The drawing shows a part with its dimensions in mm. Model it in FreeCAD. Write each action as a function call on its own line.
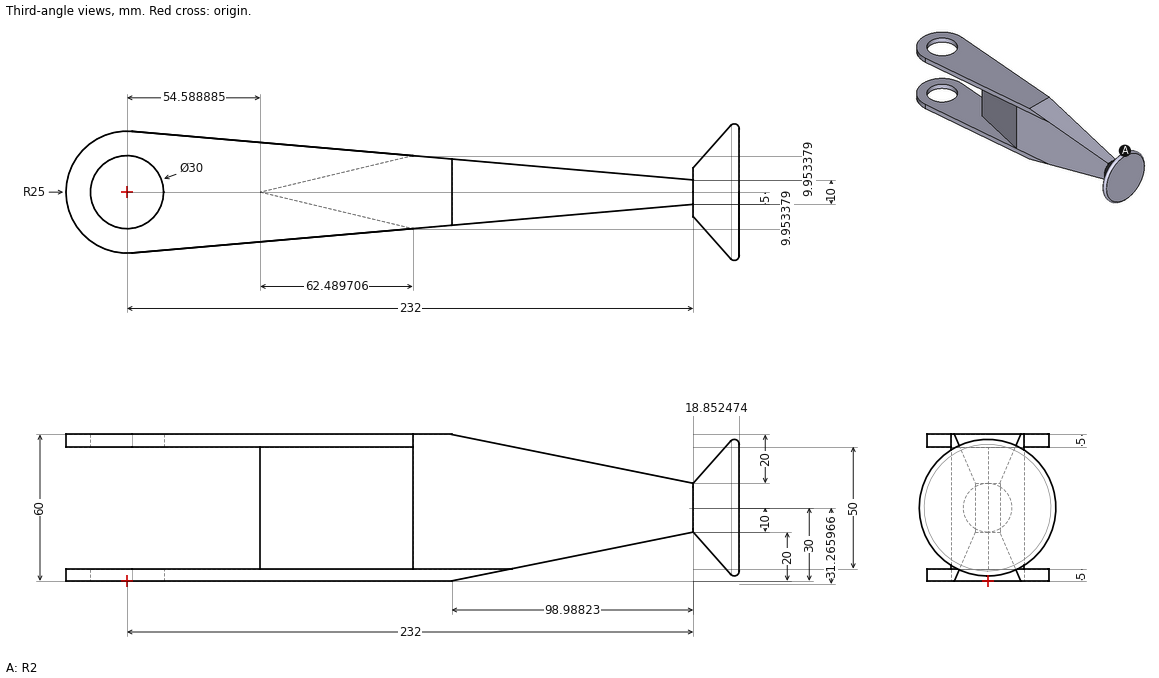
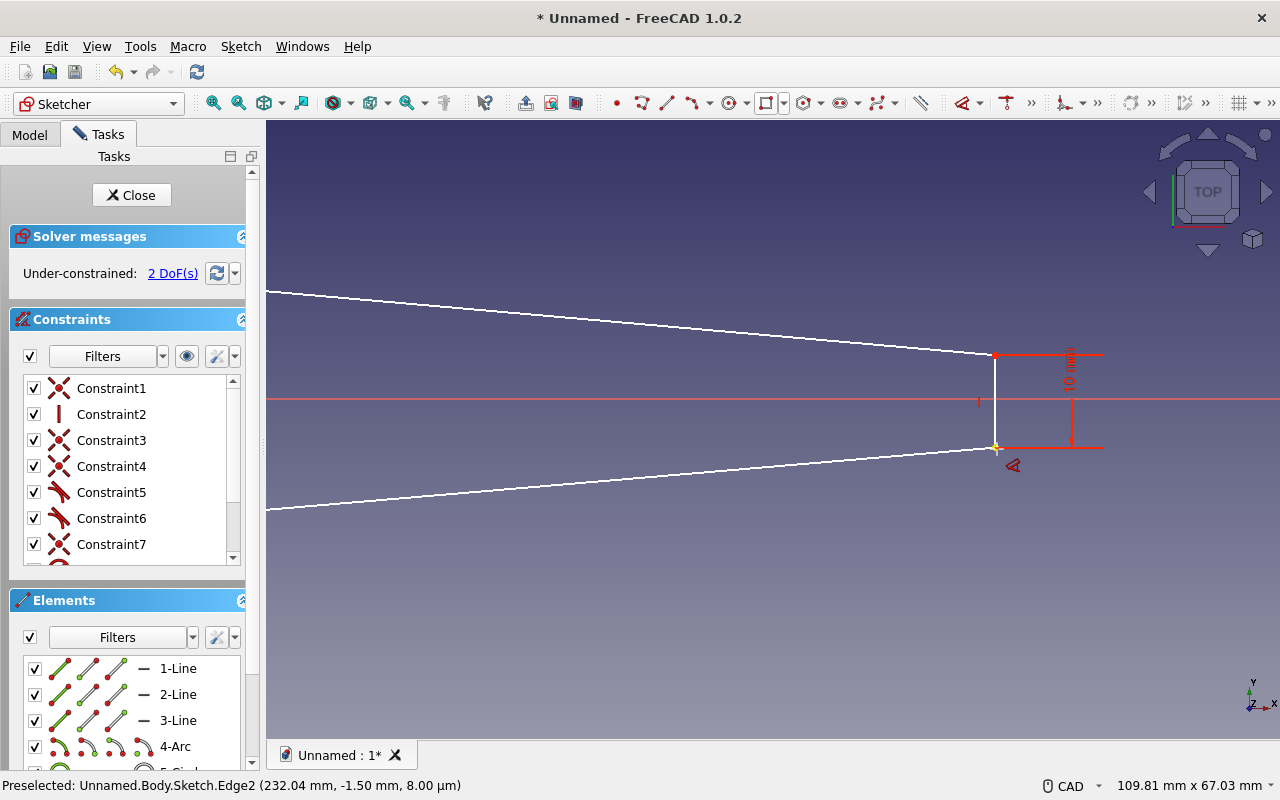
click(995, 448)
click(1029, 423)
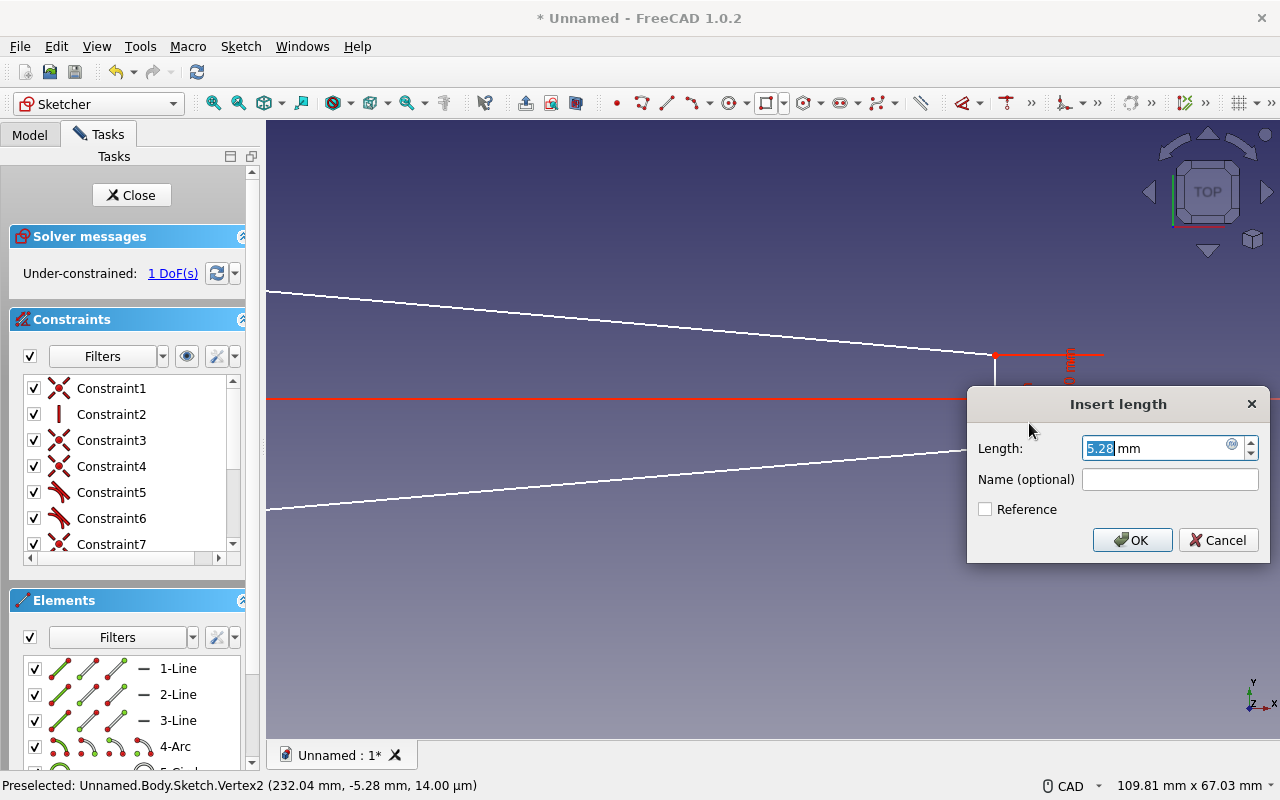
text(5)
key(Return)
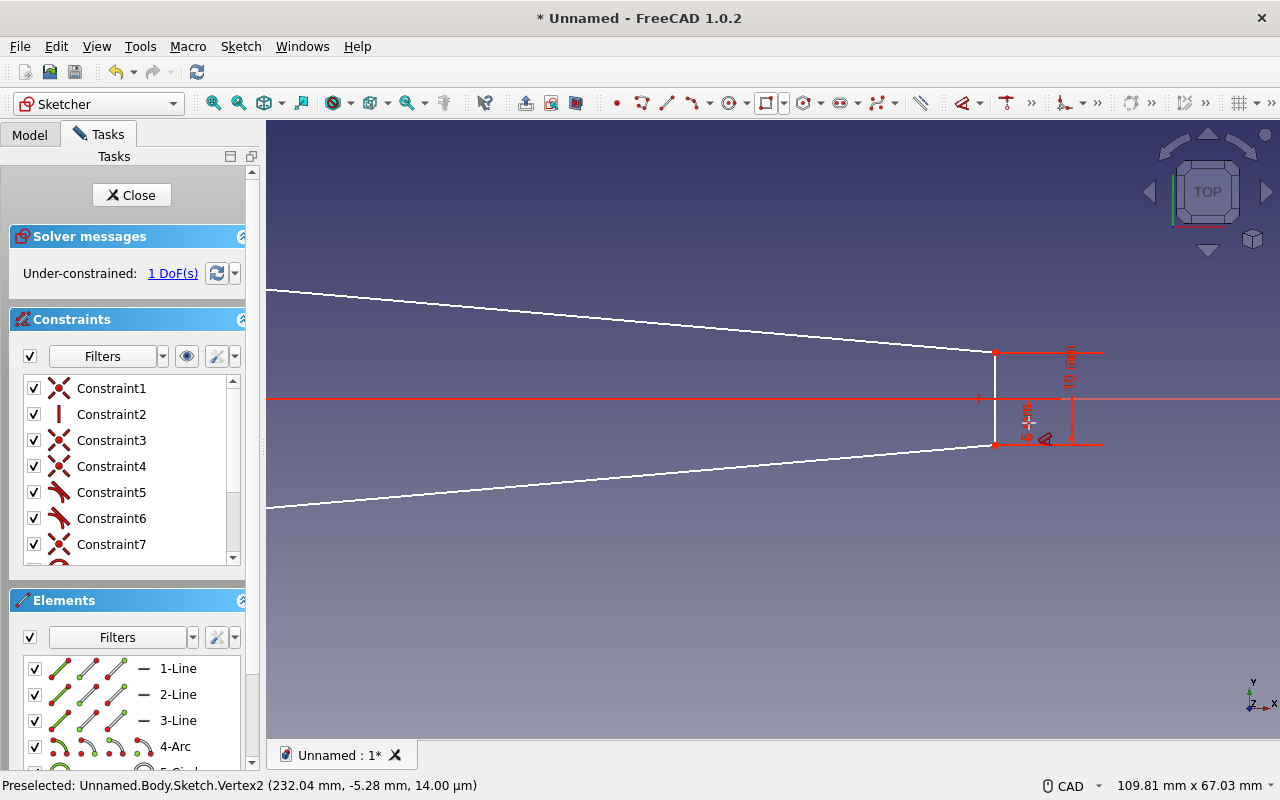
scroll(998, 440, down, 7)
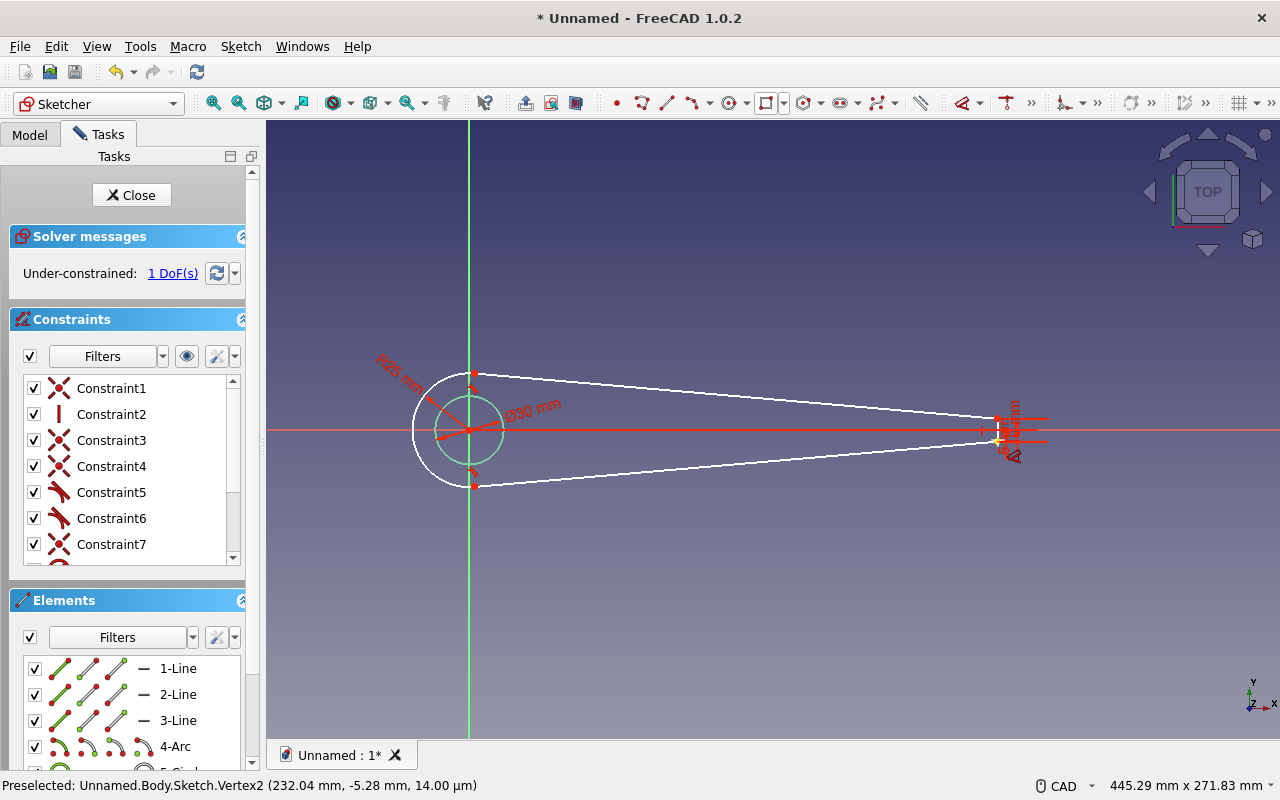
click(998, 442)
click(855, 476)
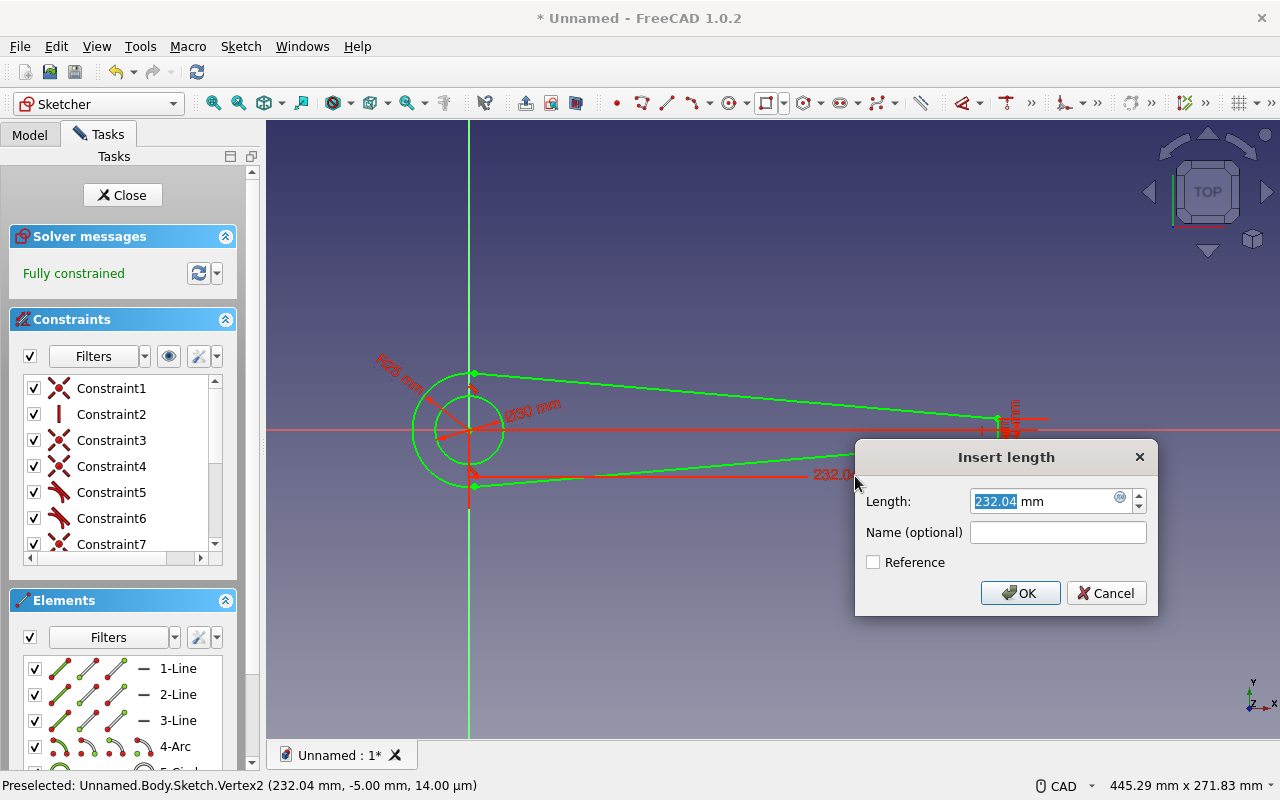
text(232)
key(Return)
key(Escape)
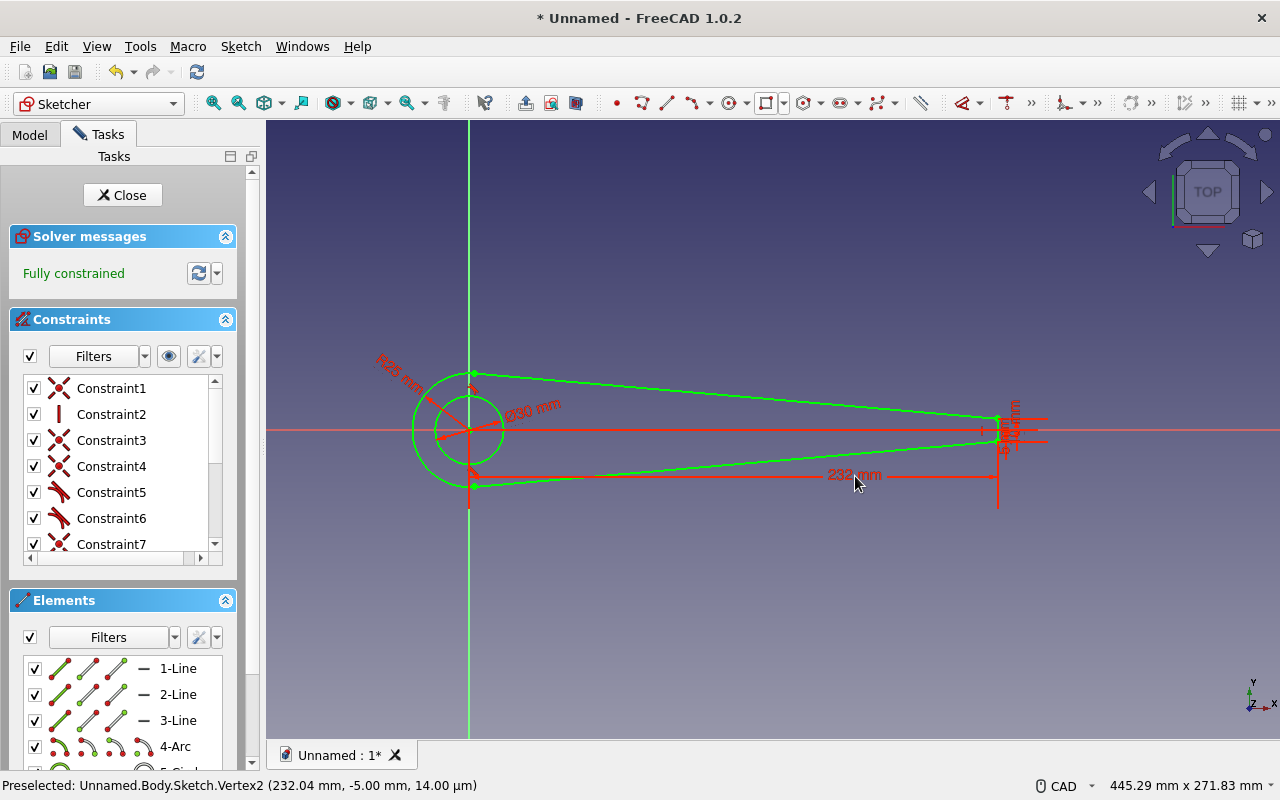
click(123, 195)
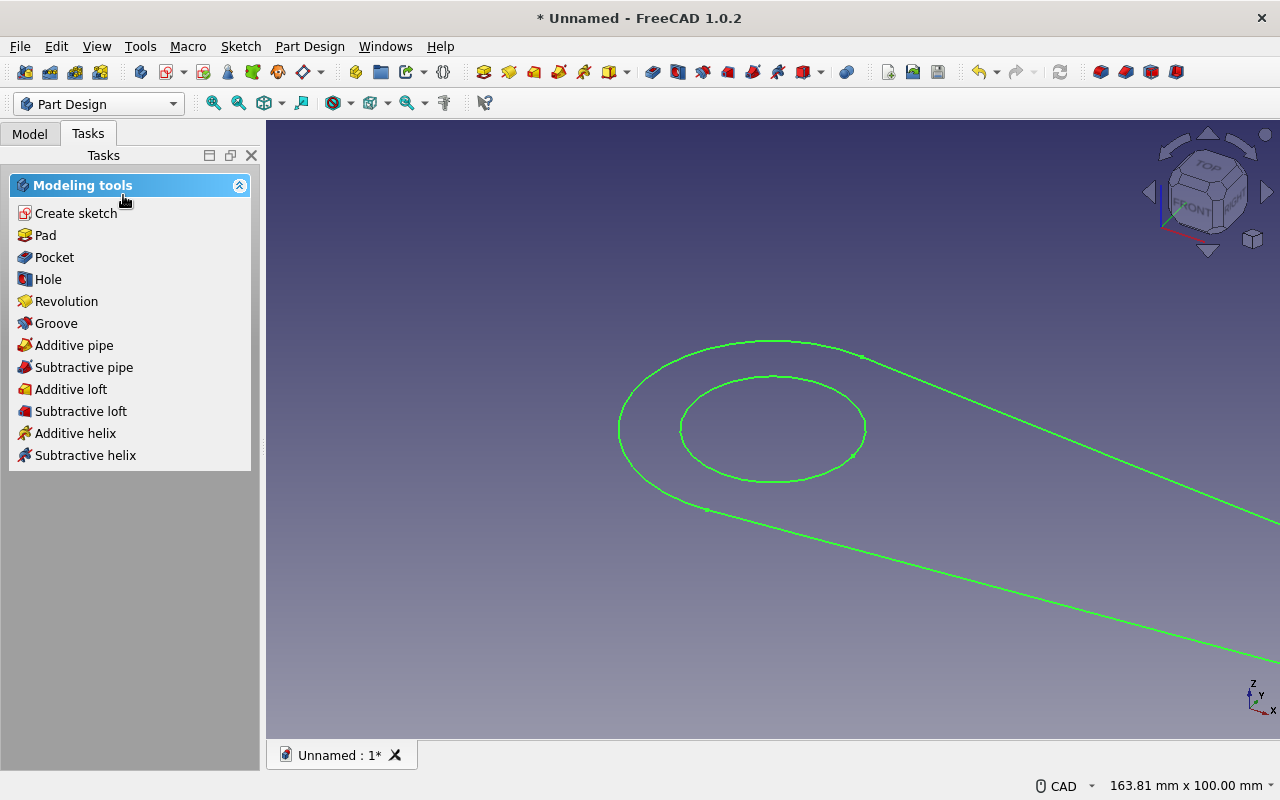
click(484, 72)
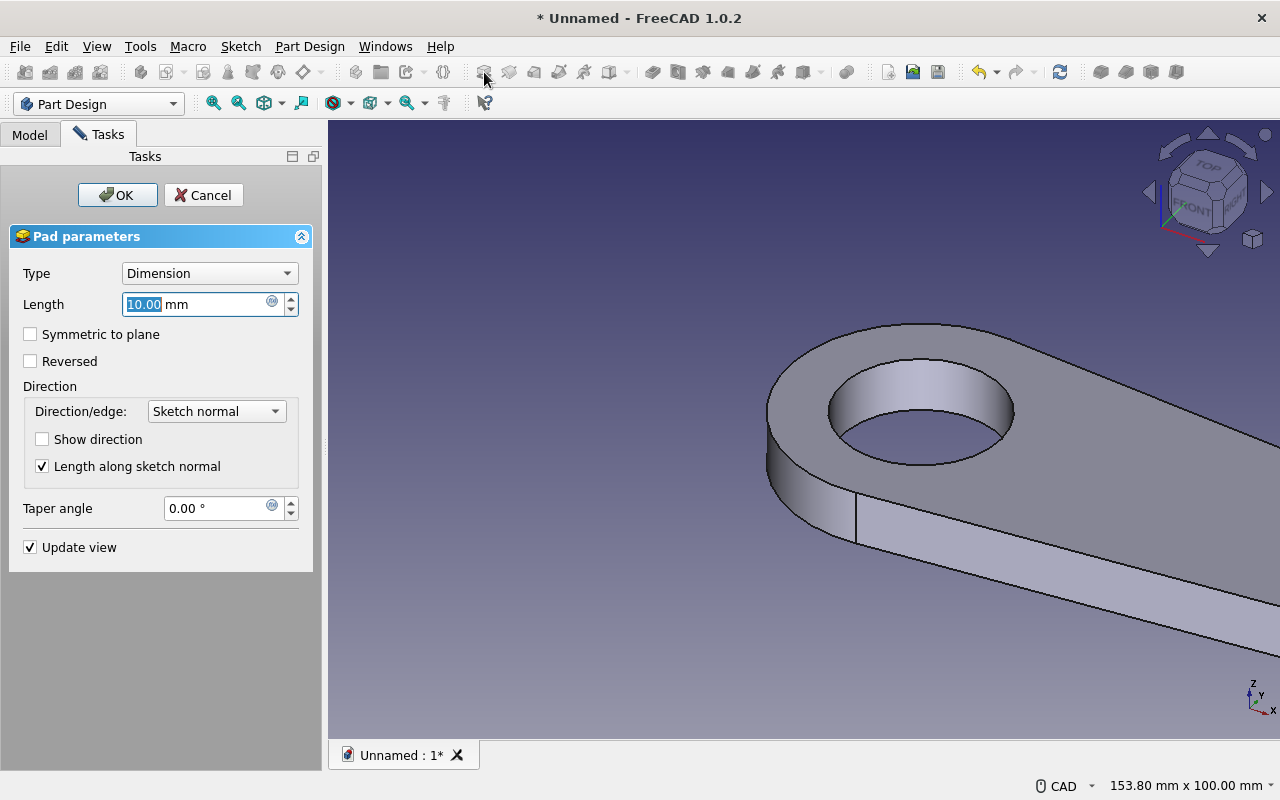
text(5)
key(Tab)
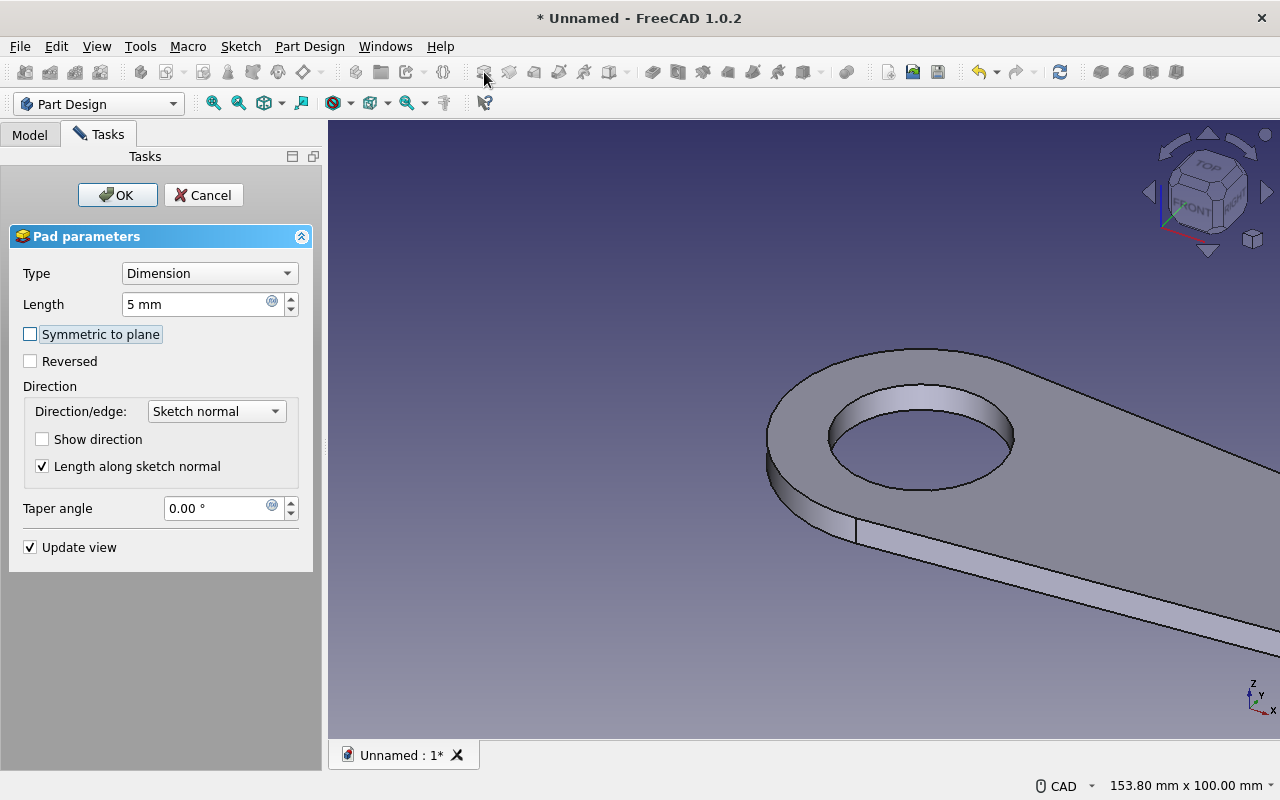
click(118, 195)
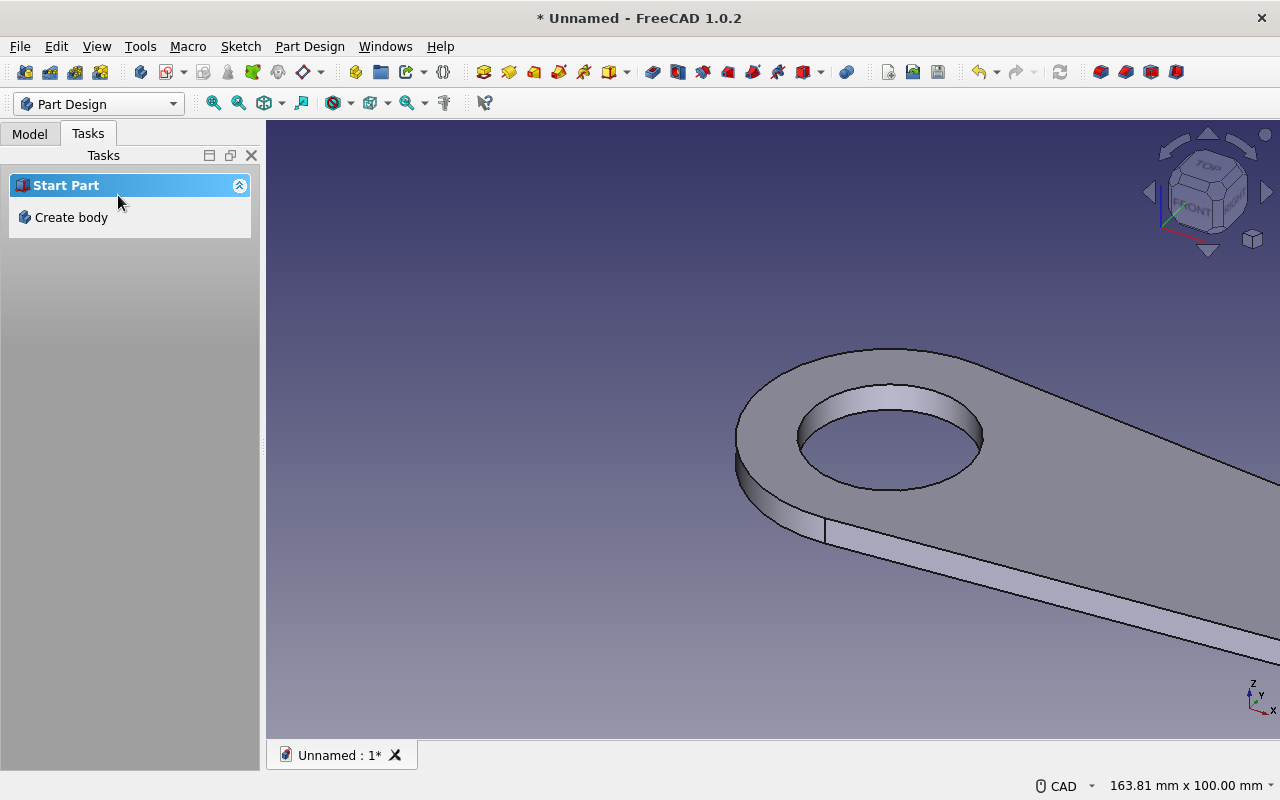
click(214, 104)